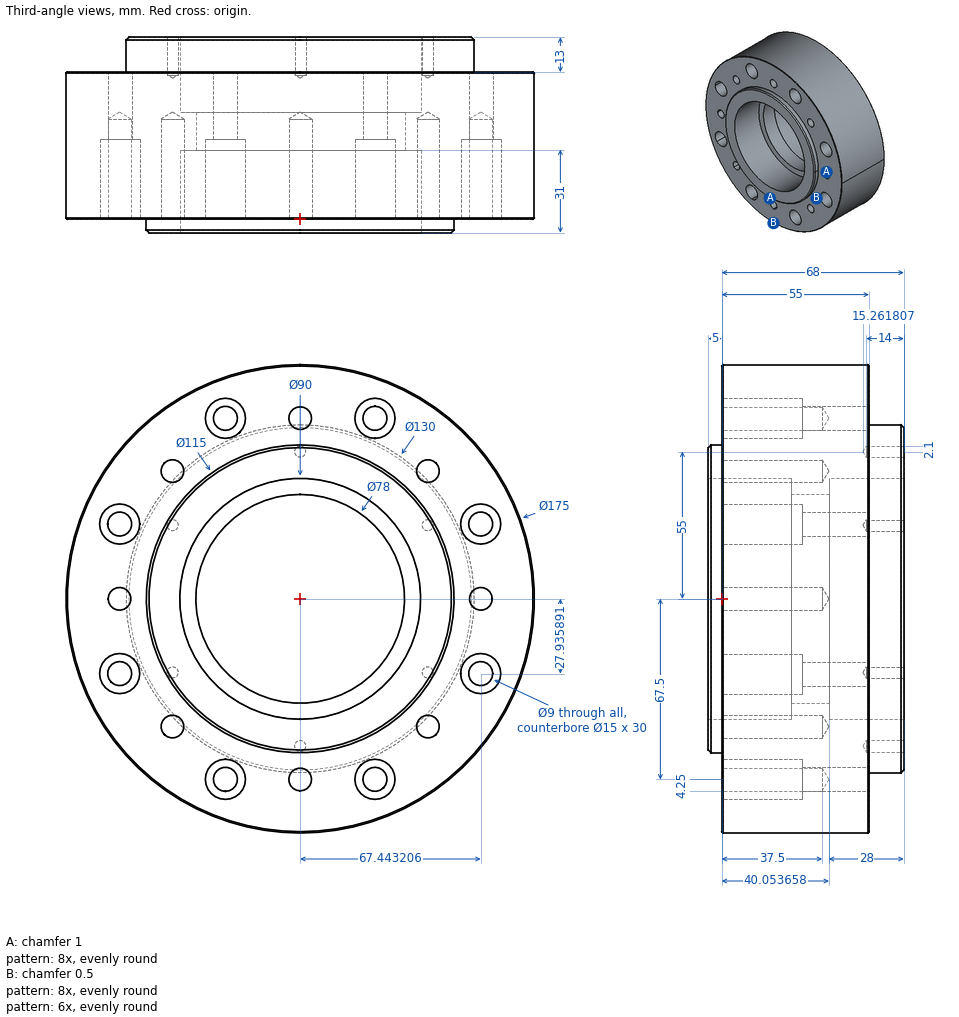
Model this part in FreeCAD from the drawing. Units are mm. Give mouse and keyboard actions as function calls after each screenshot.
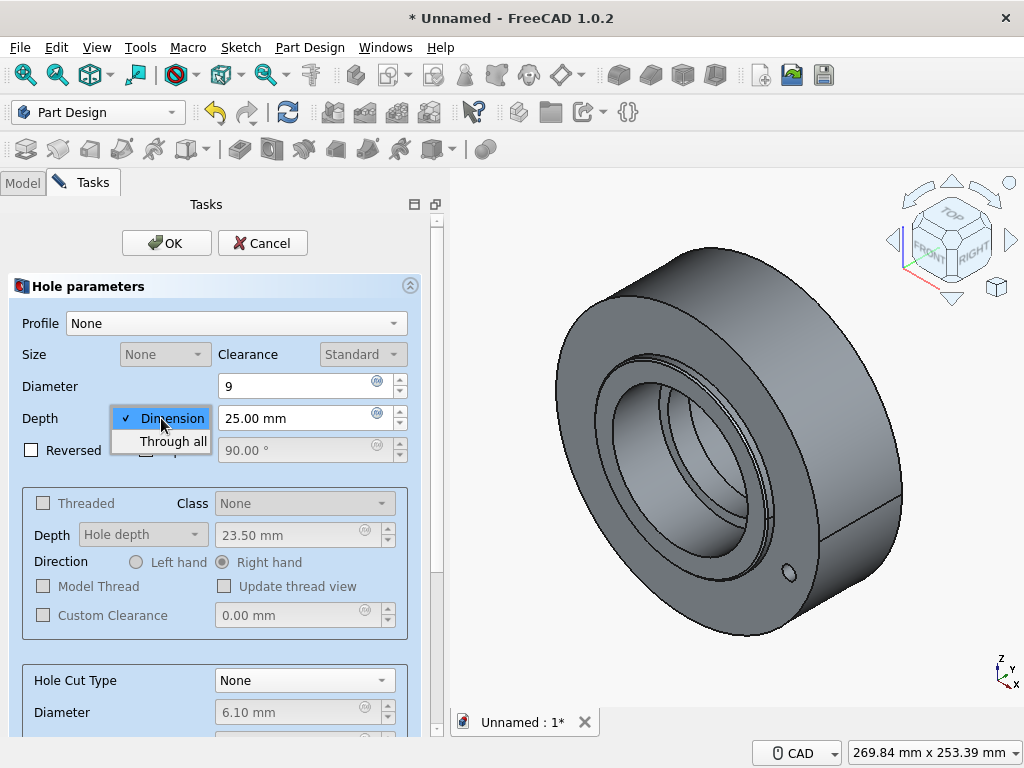
click(160, 442)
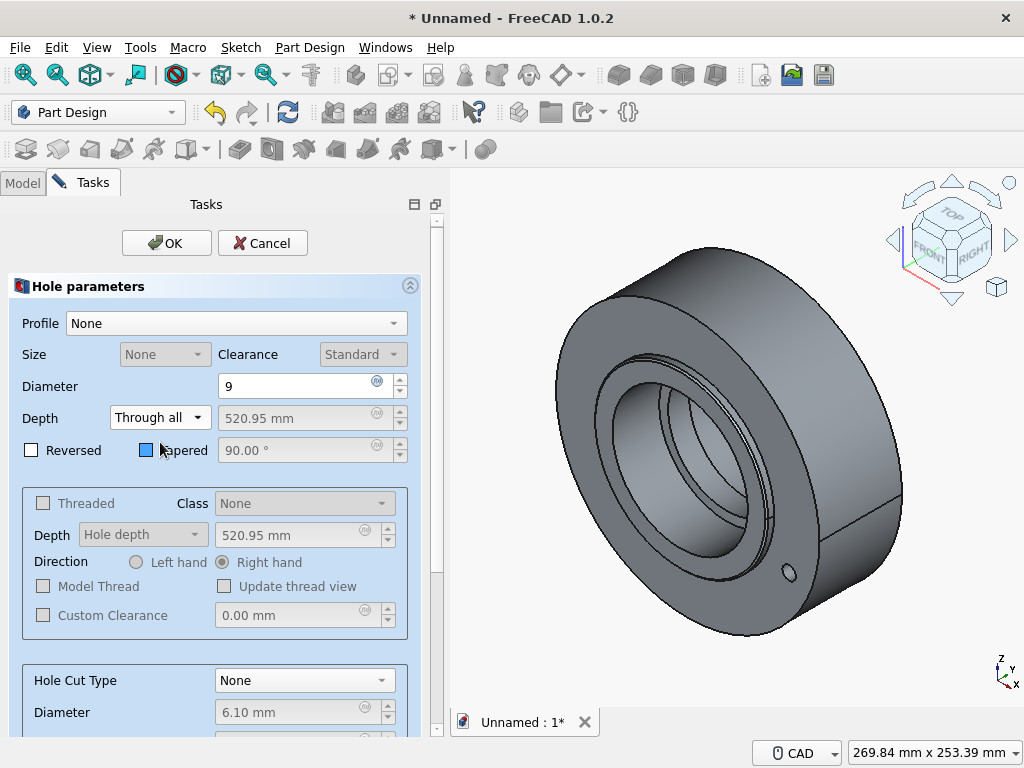
click(306, 680)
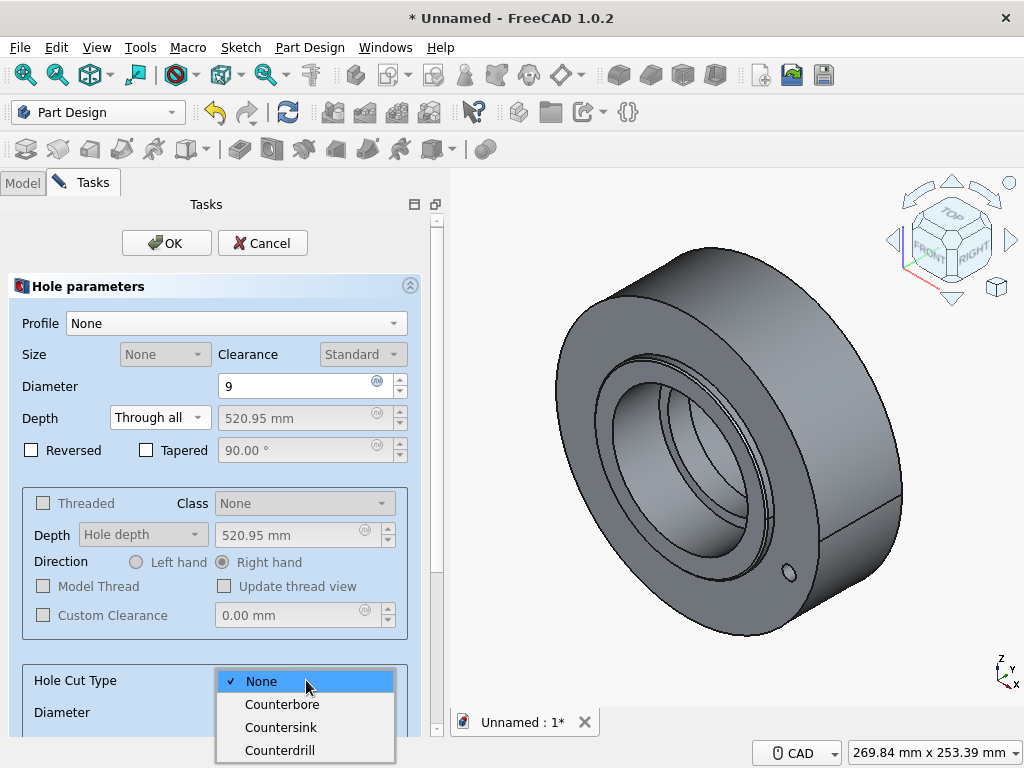
click(304, 704)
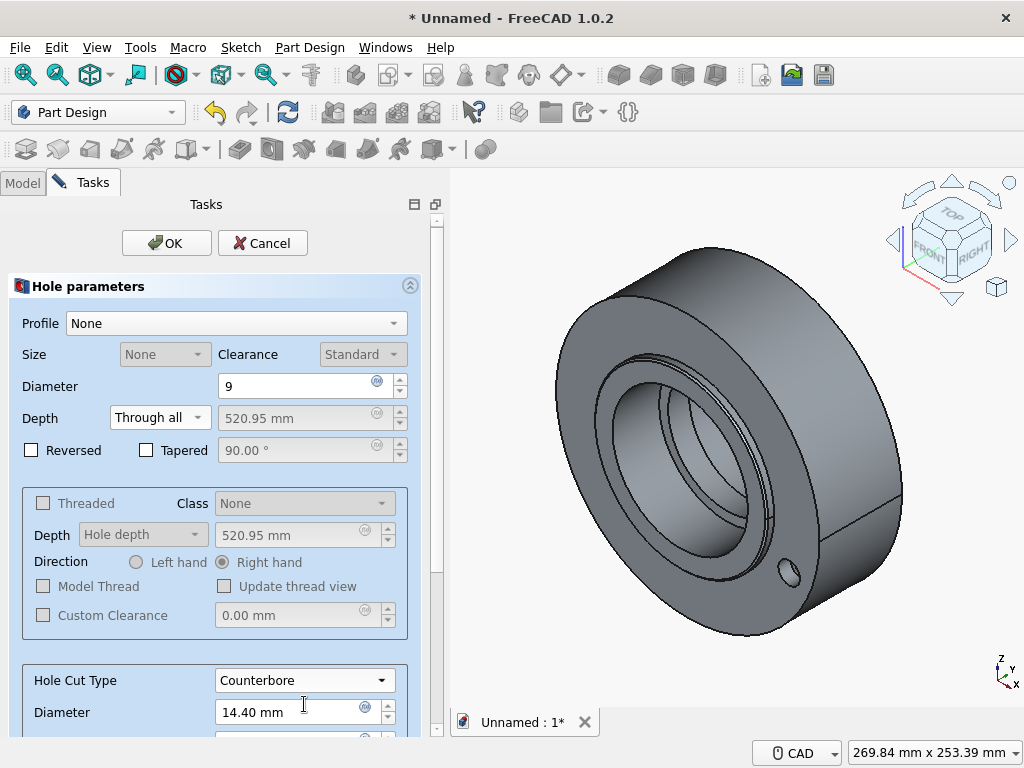
triple_click(298, 712)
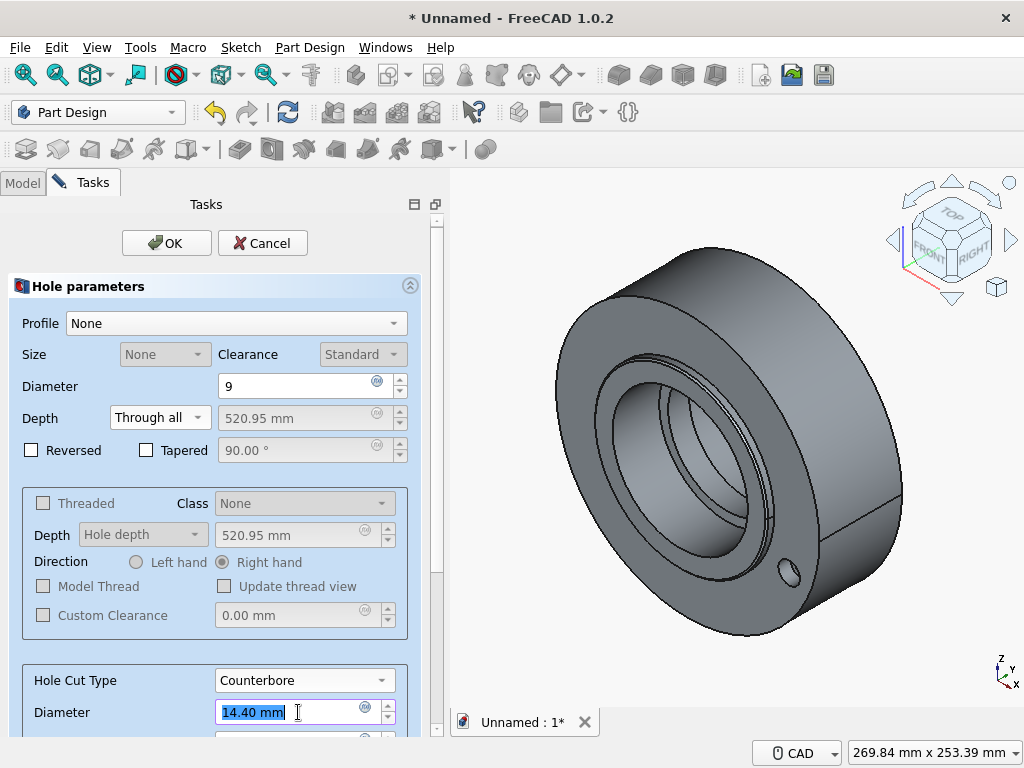
text(15)
key(Tab)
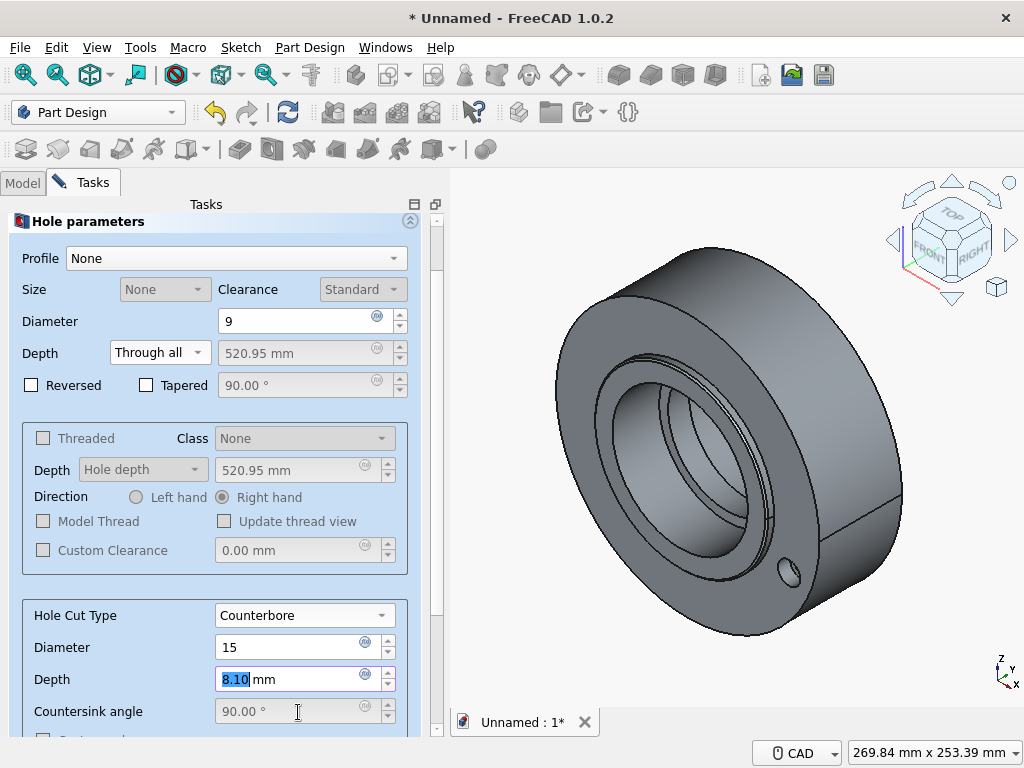
text(30)
key(Tab)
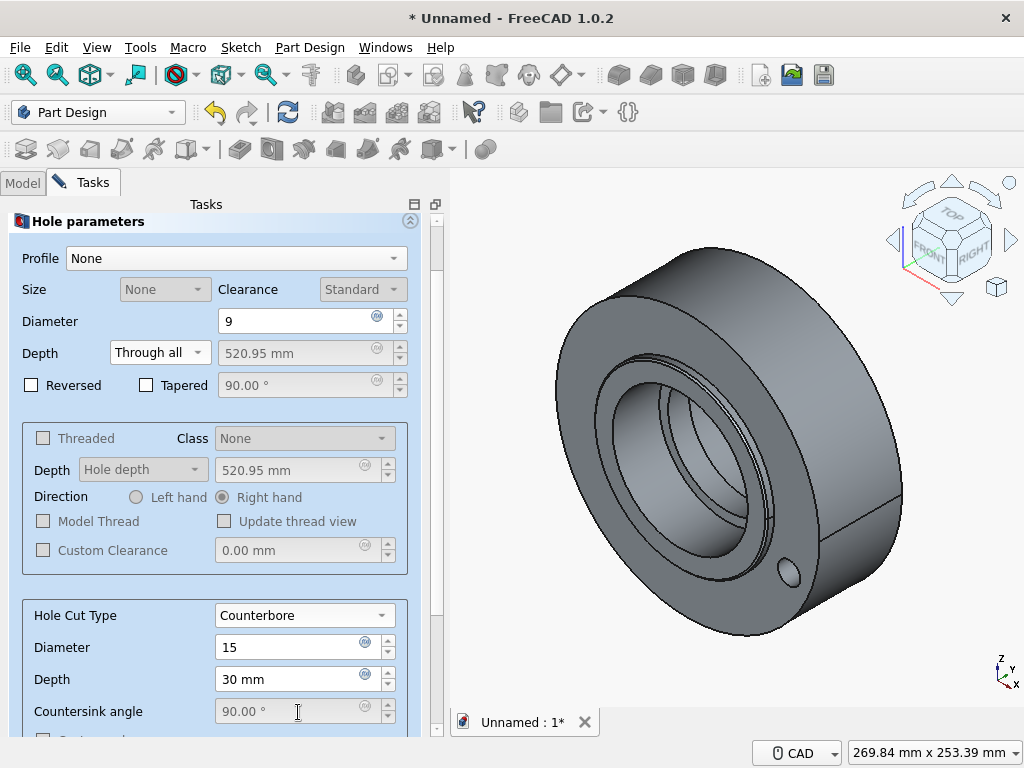
scroll(437, 475, up, 2)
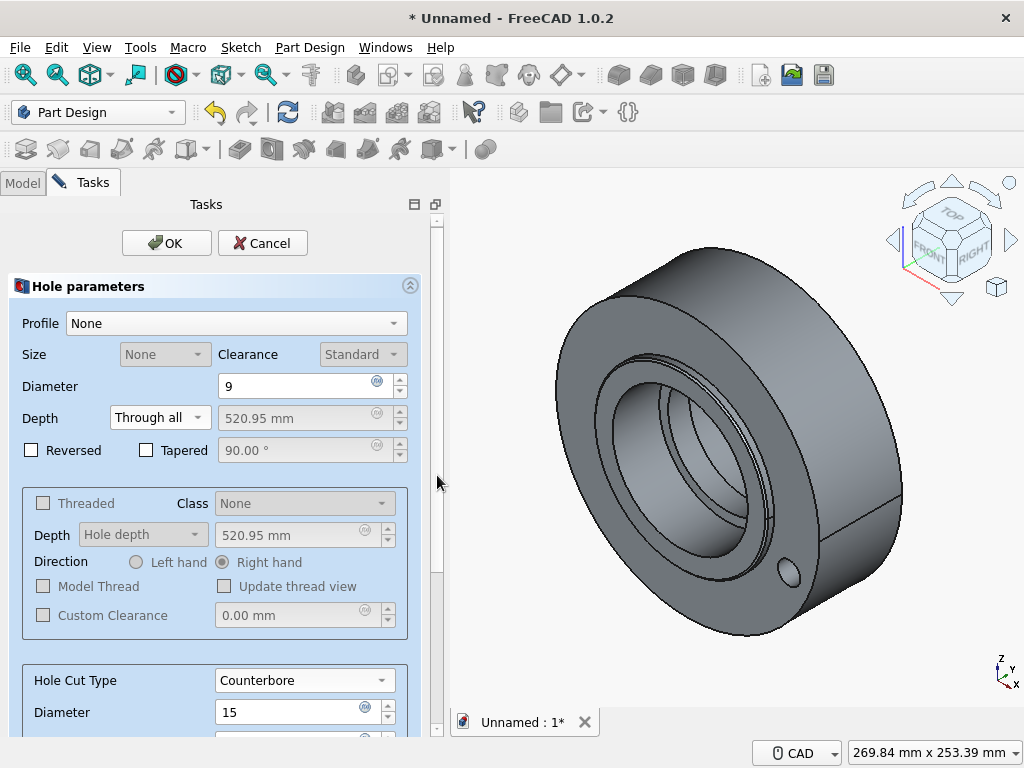
click(167, 243)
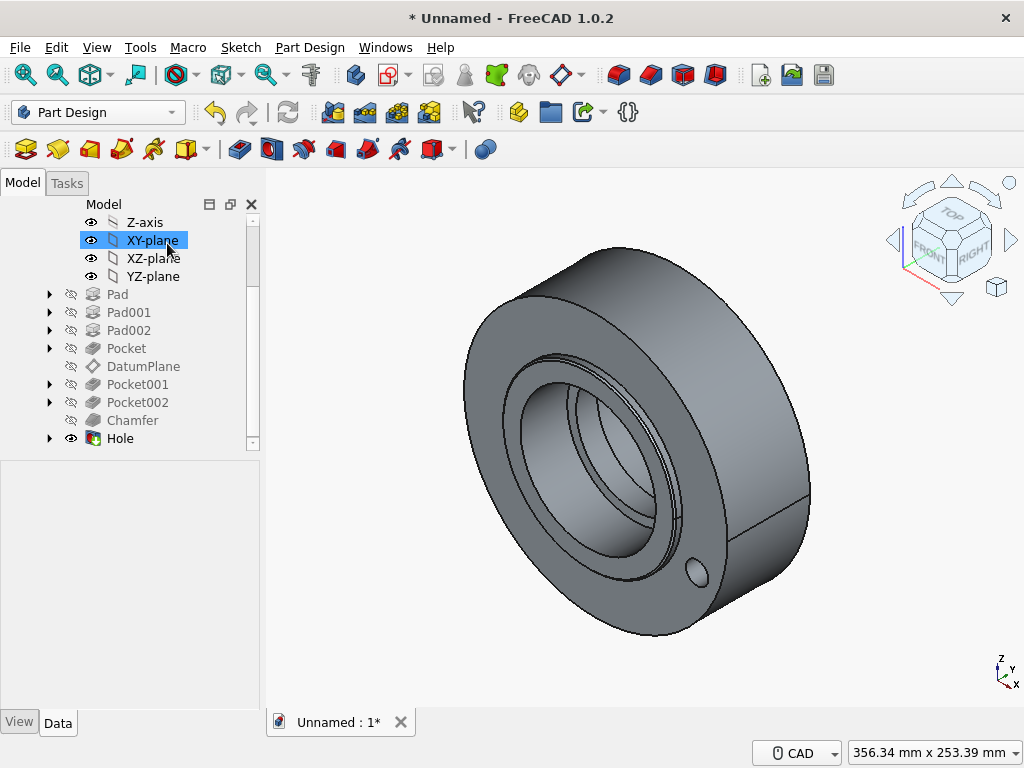
click(116, 438)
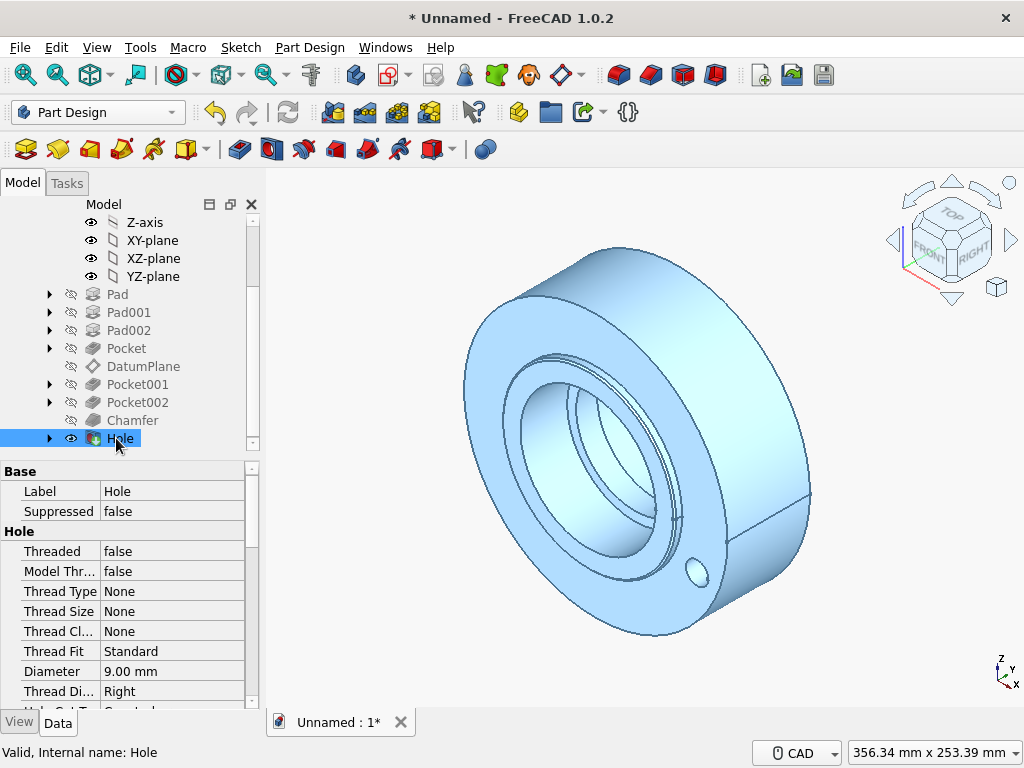
click(398, 112)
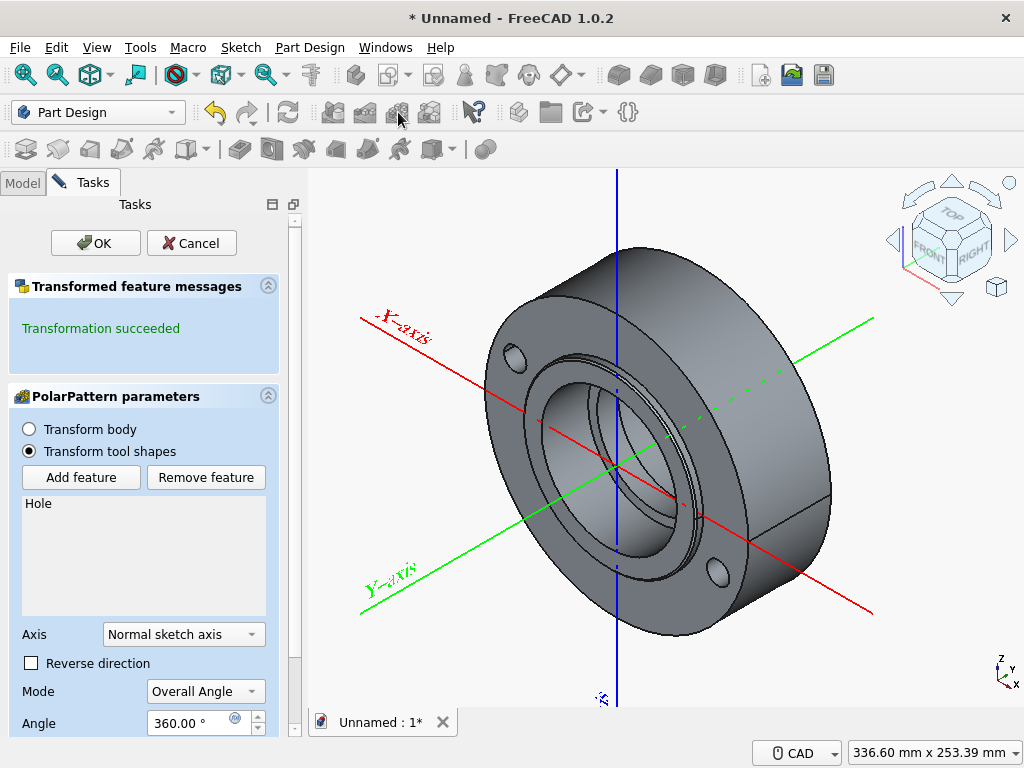
click(184, 634)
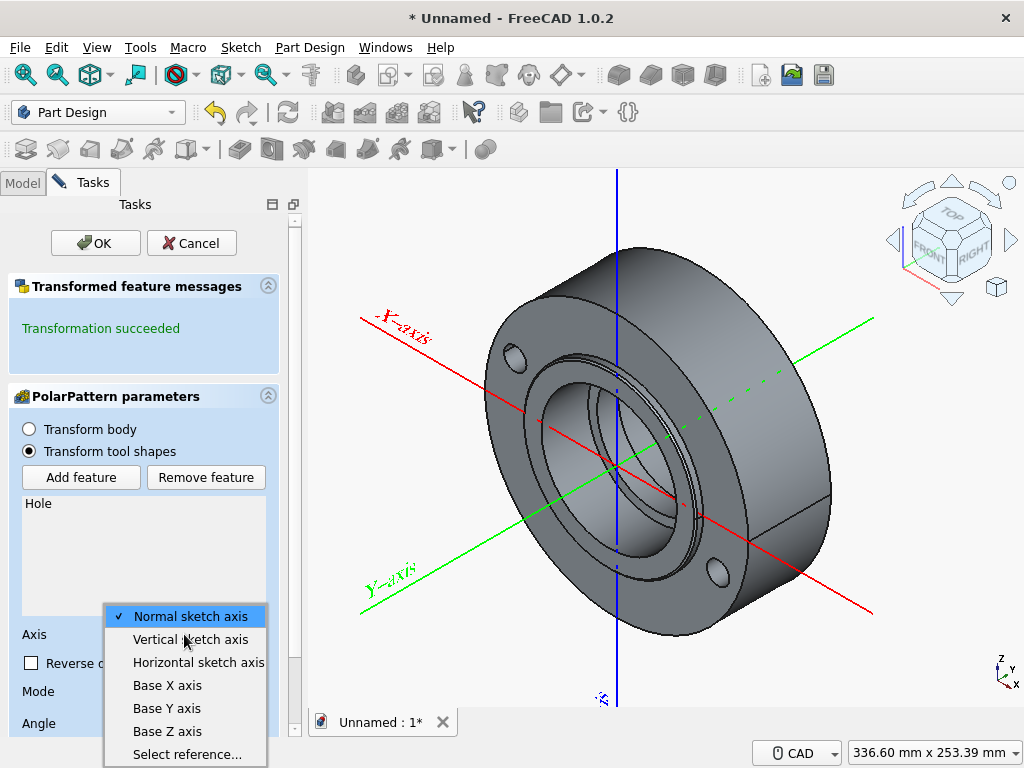
click(184, 708)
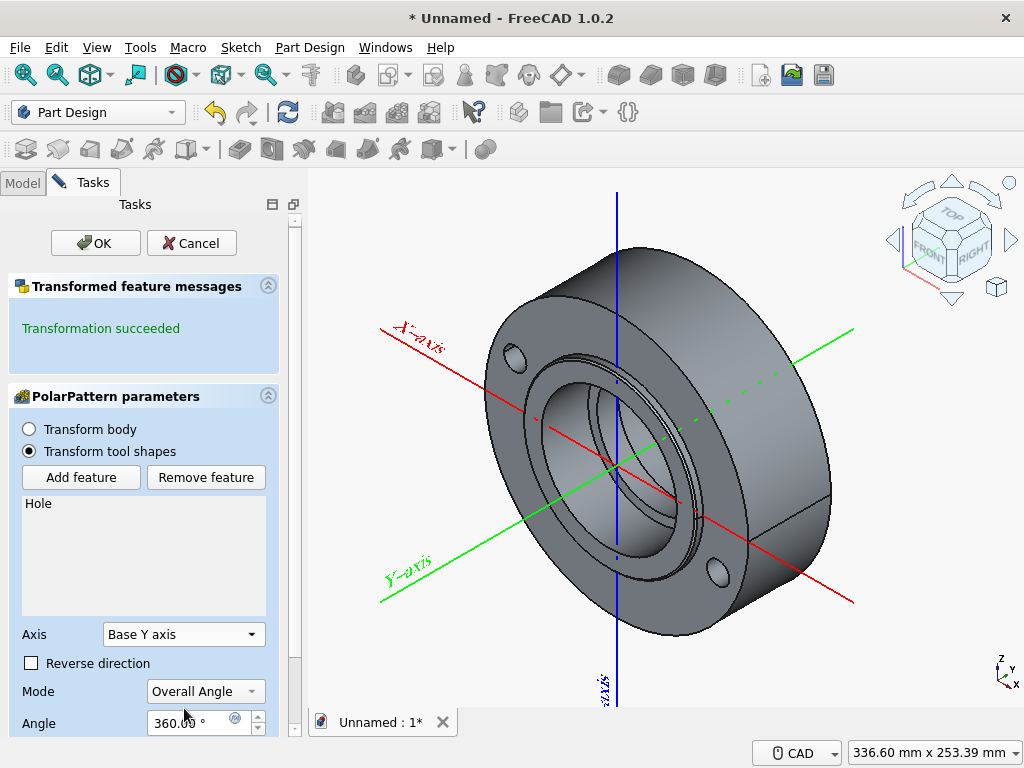
scroll(295, 475, down, 2)